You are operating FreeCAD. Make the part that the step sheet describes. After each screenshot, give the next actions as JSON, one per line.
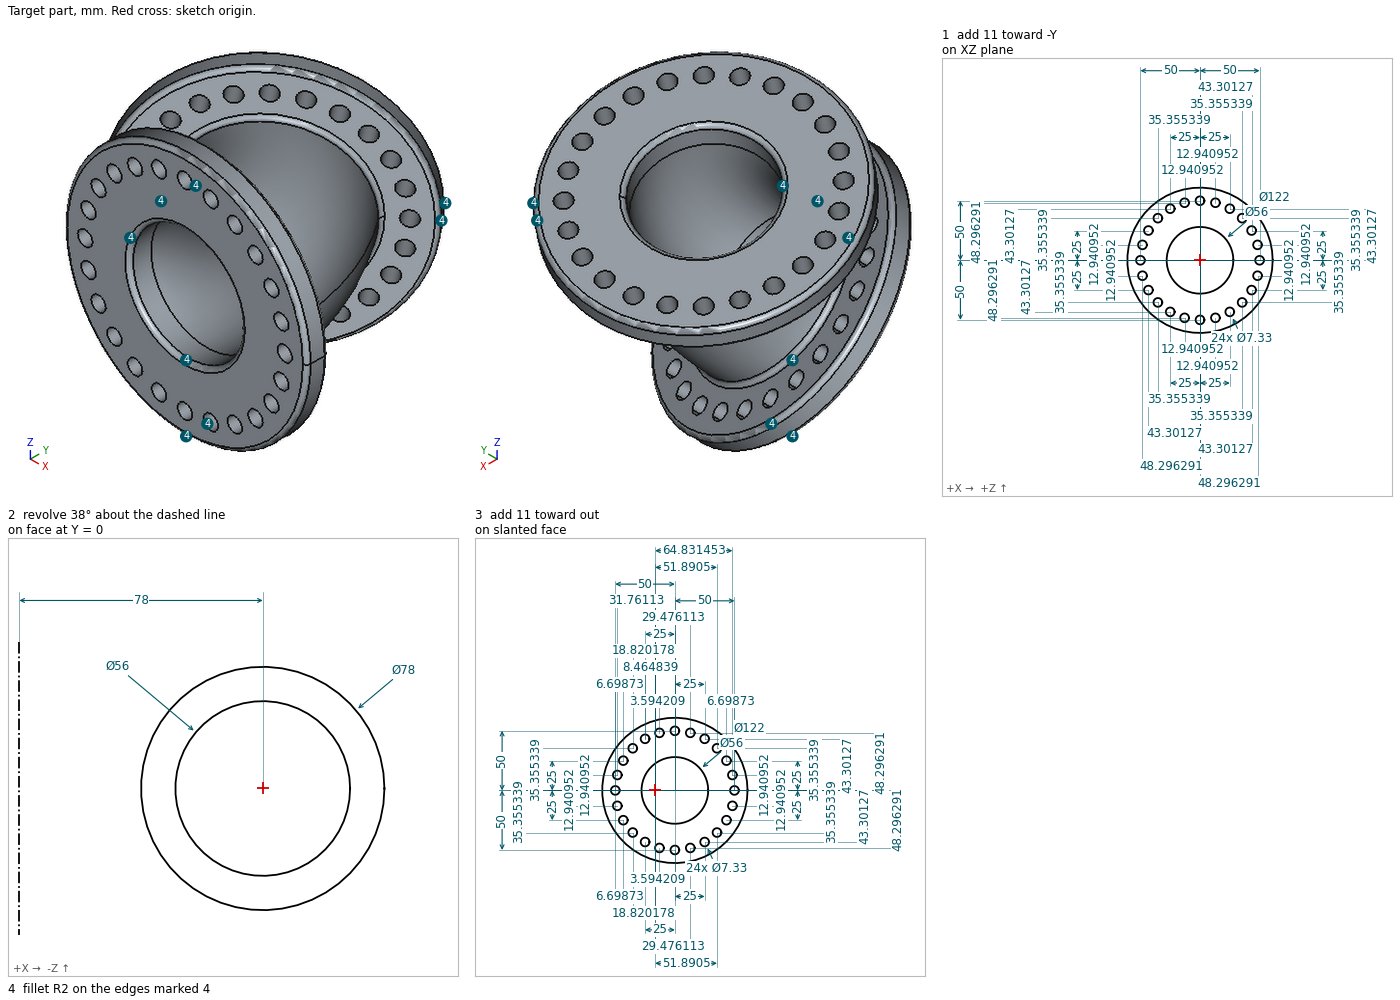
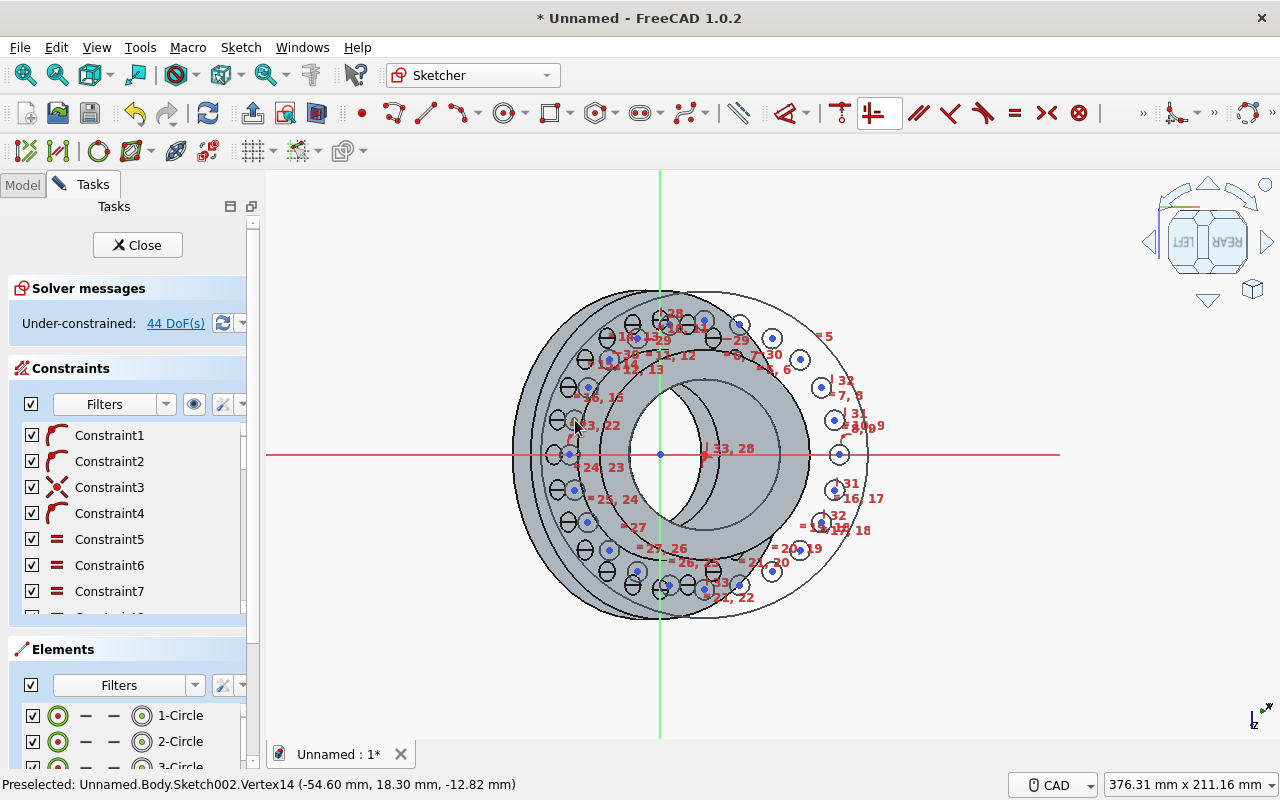
{"action": "left_click", "coordinate": [575, 490]}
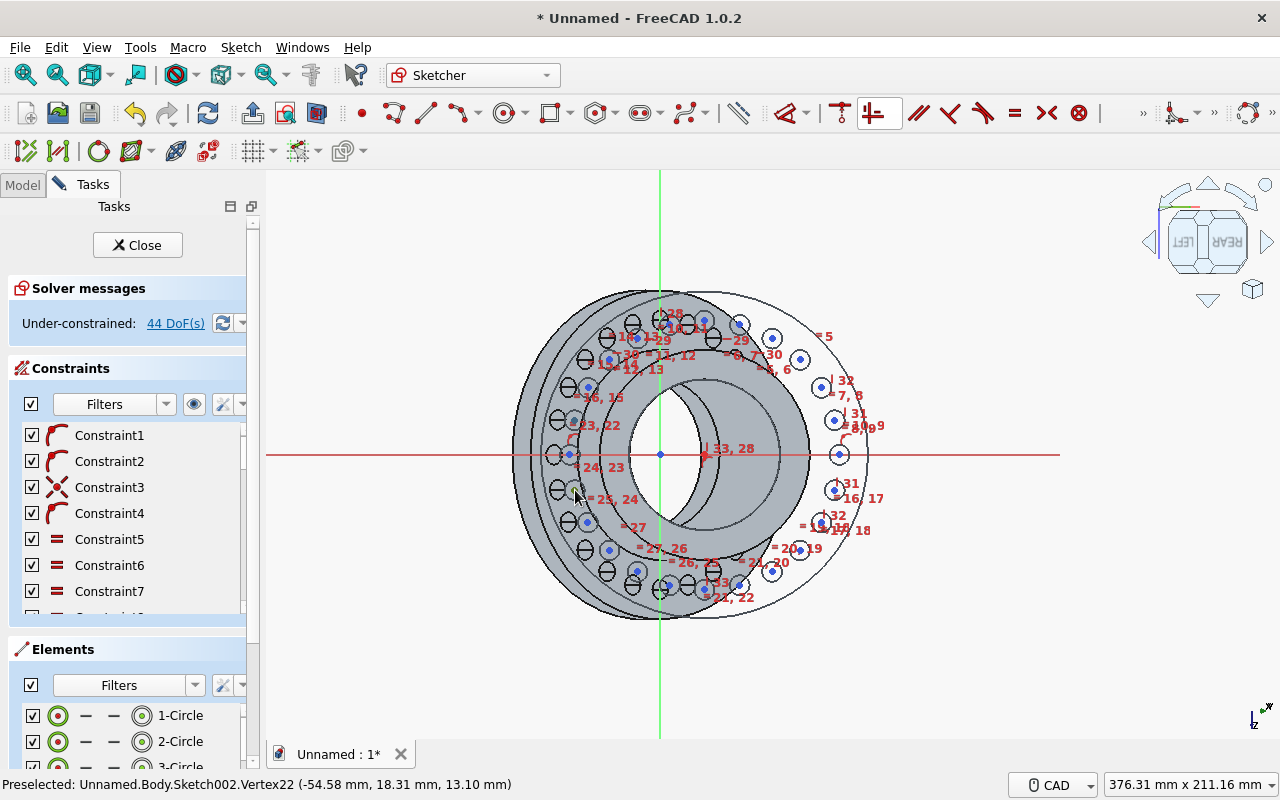
{"action": "key", "text": "v"}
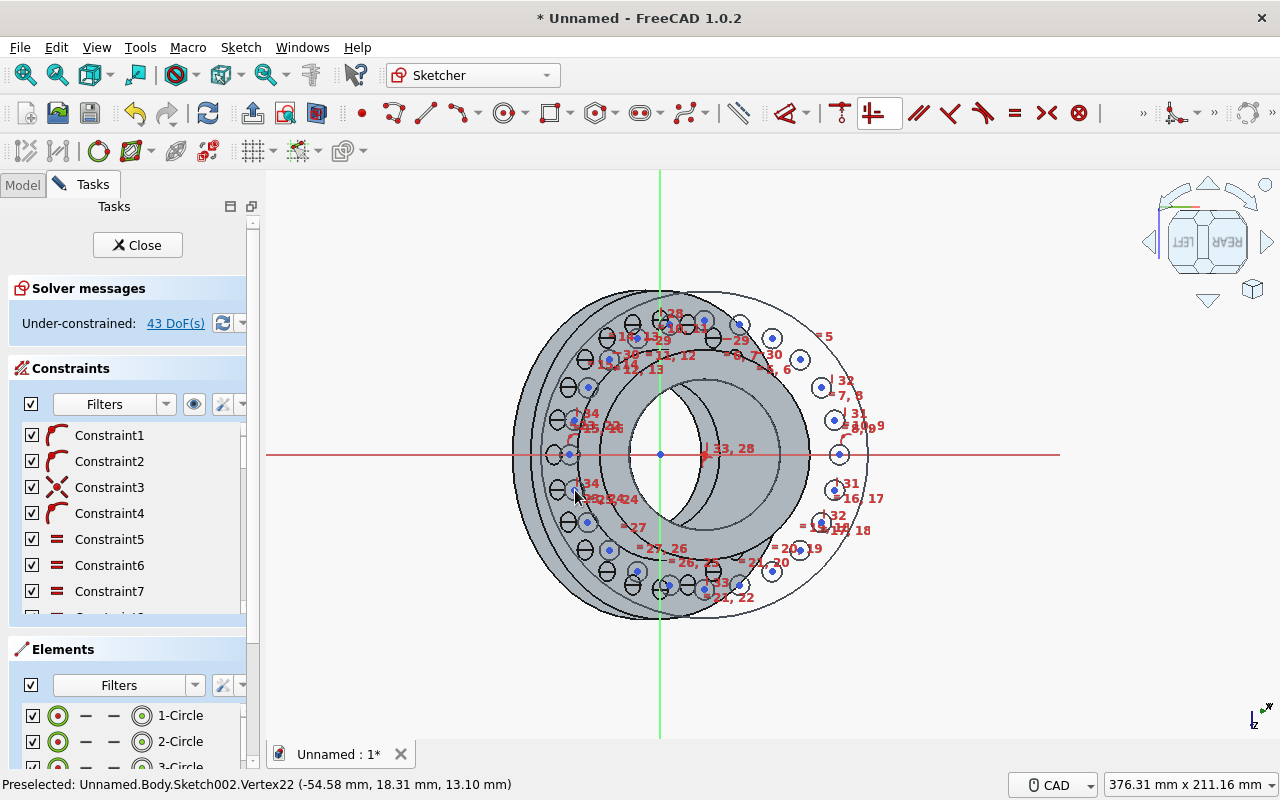
{"action": "scroll", "coordinate": [740, 585], "scroll_direction": "up", "scroll_amount": 4}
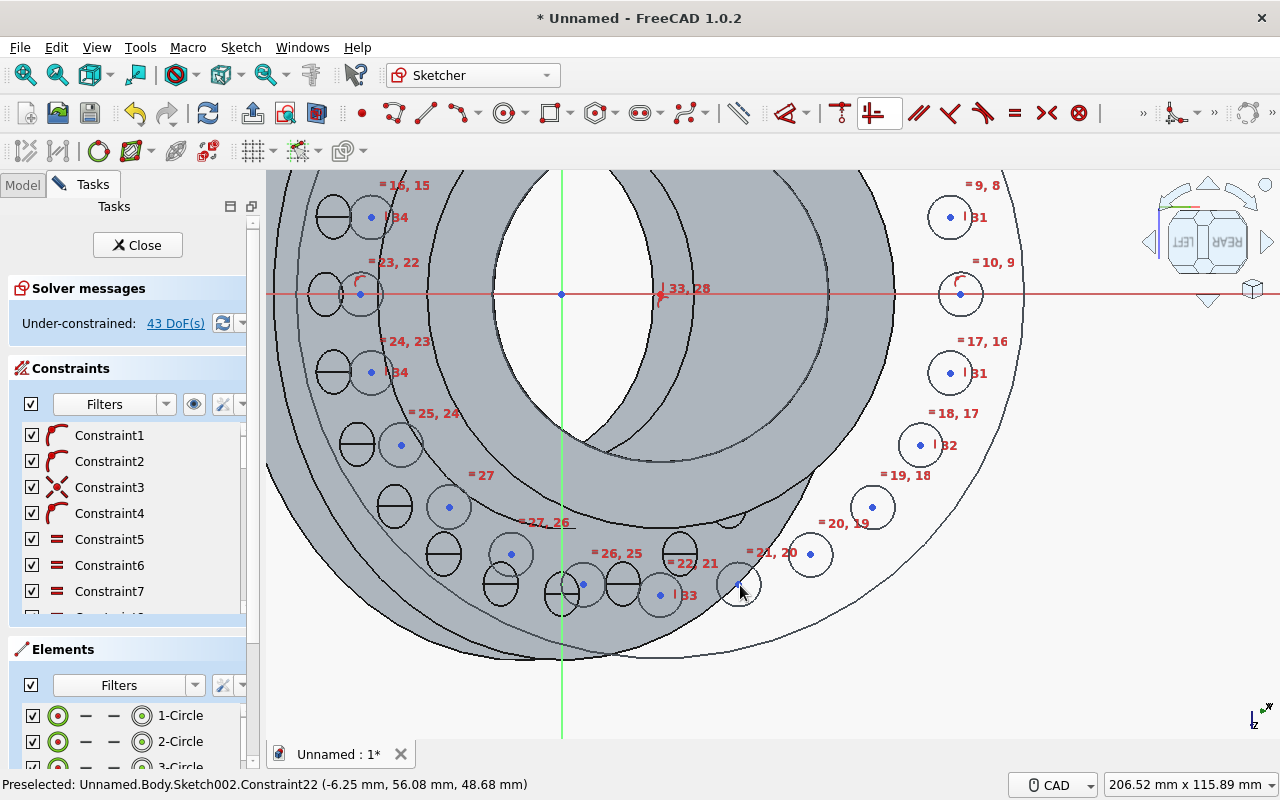
{"action": "left_click", "coordinate": [739, 584]}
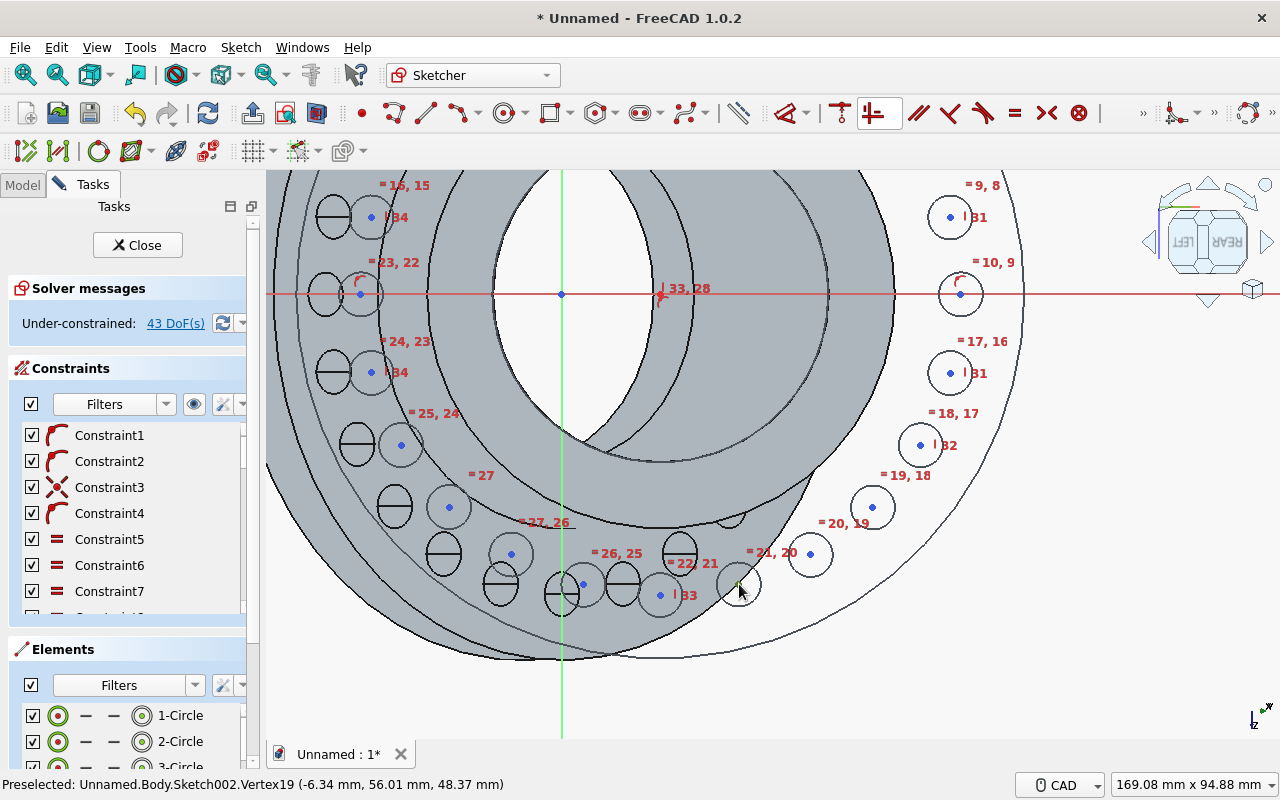
{"action": "left_click", "coordinate": [583, 585]}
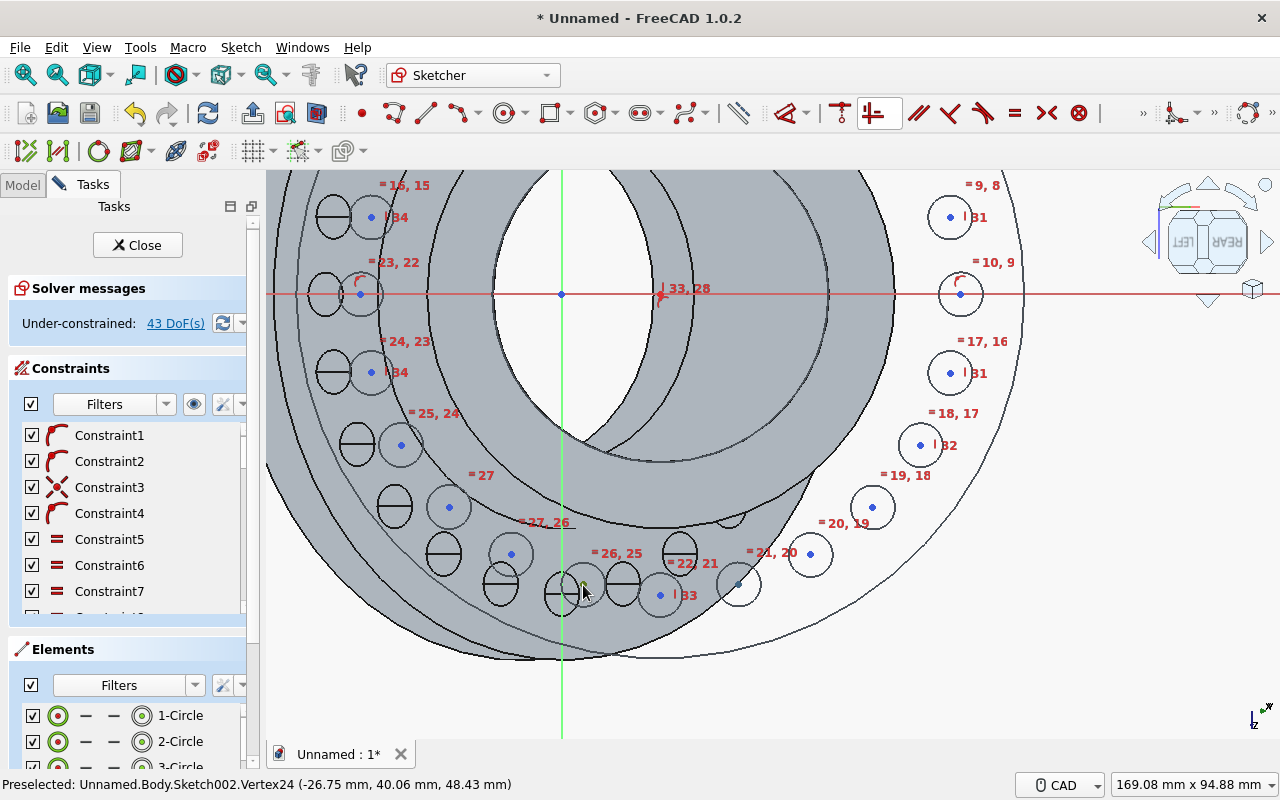
{"action": "left_click", "coordinate": [896, 114]}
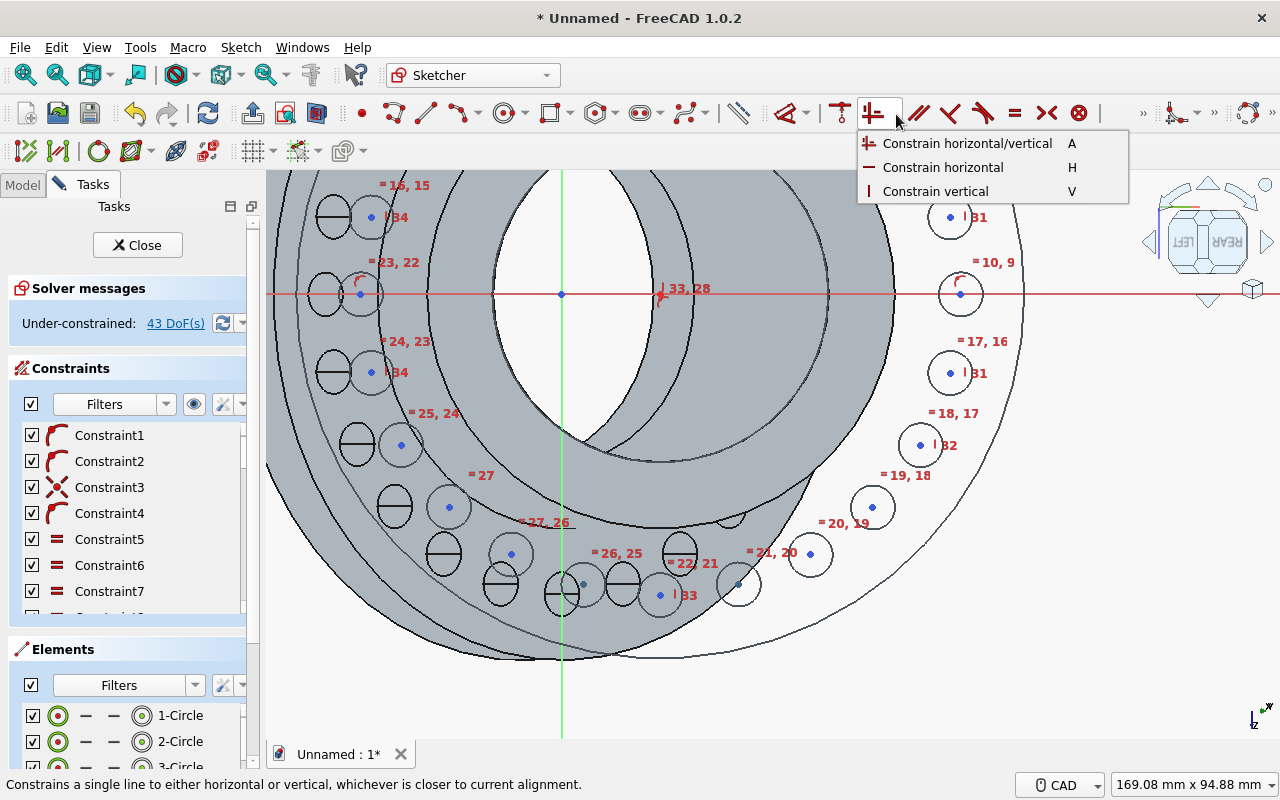
{"action": "left_click", "coordinate": [993, 167]}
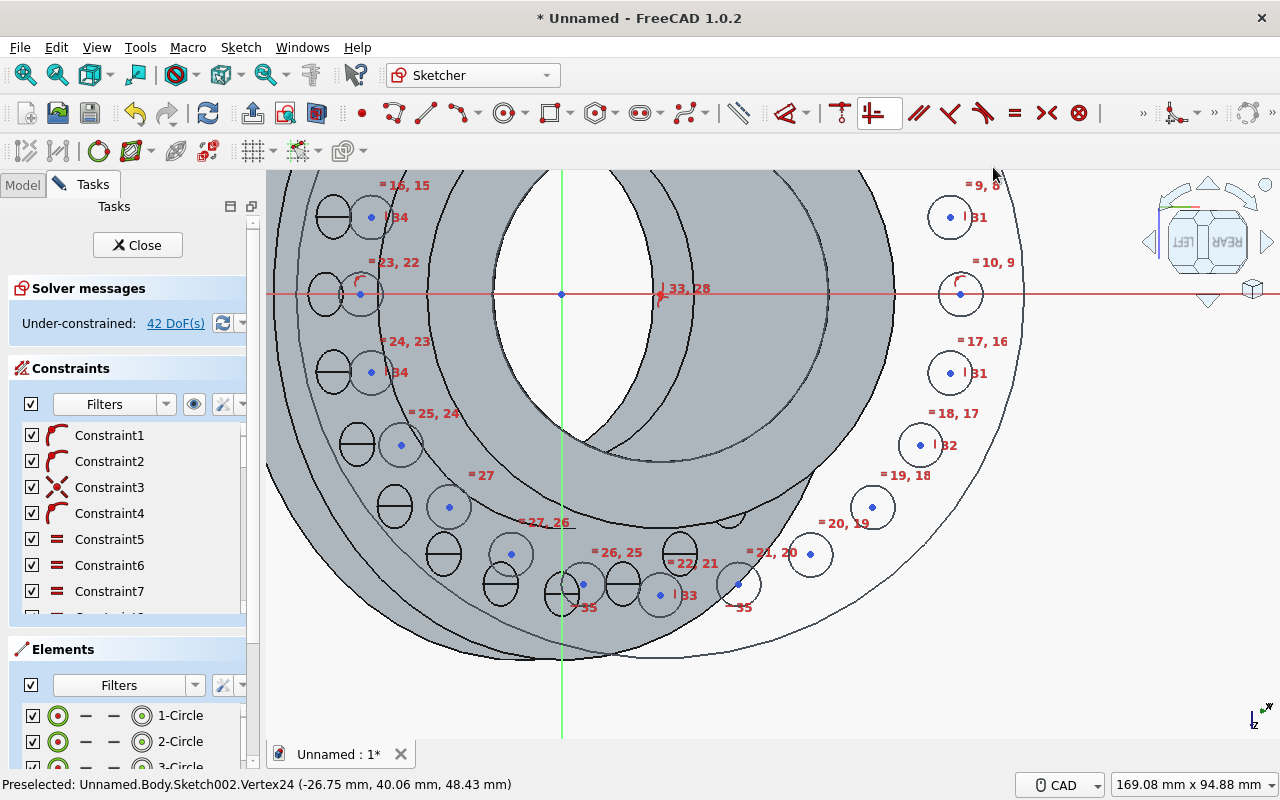
{"action": "left_click", "coordinate": [811, 555]}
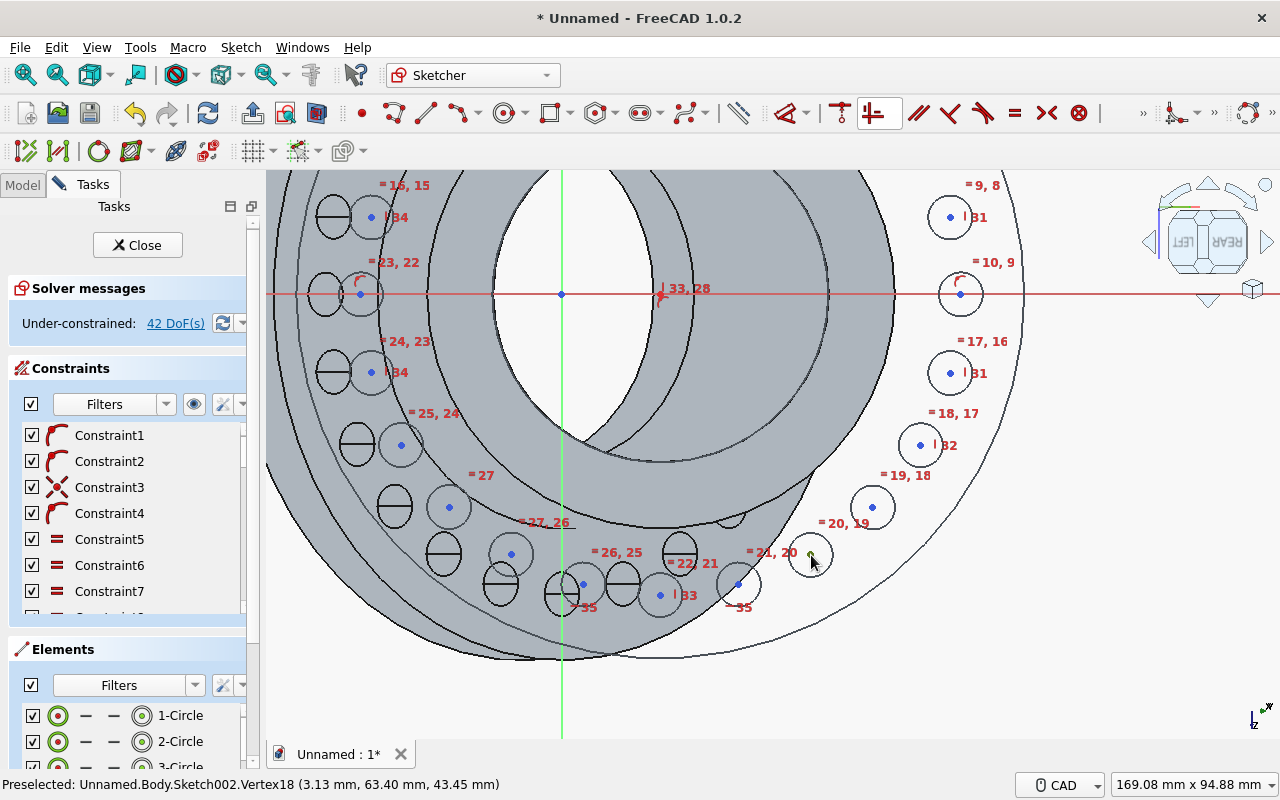
{"action": "left_click", "coordinate": [511, 555]}